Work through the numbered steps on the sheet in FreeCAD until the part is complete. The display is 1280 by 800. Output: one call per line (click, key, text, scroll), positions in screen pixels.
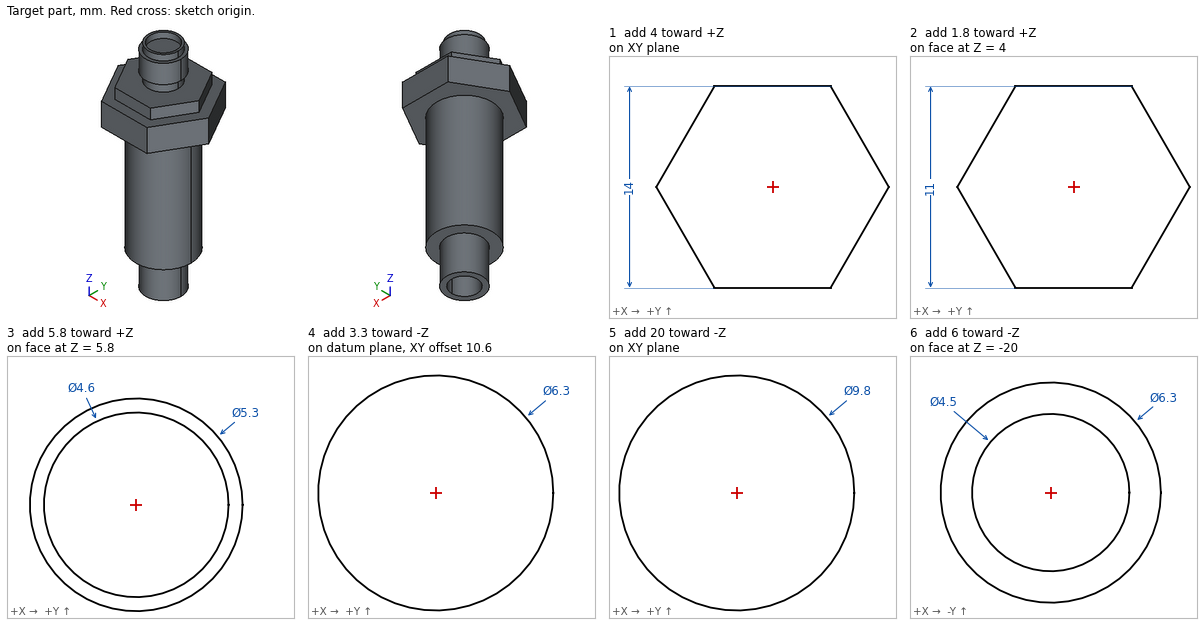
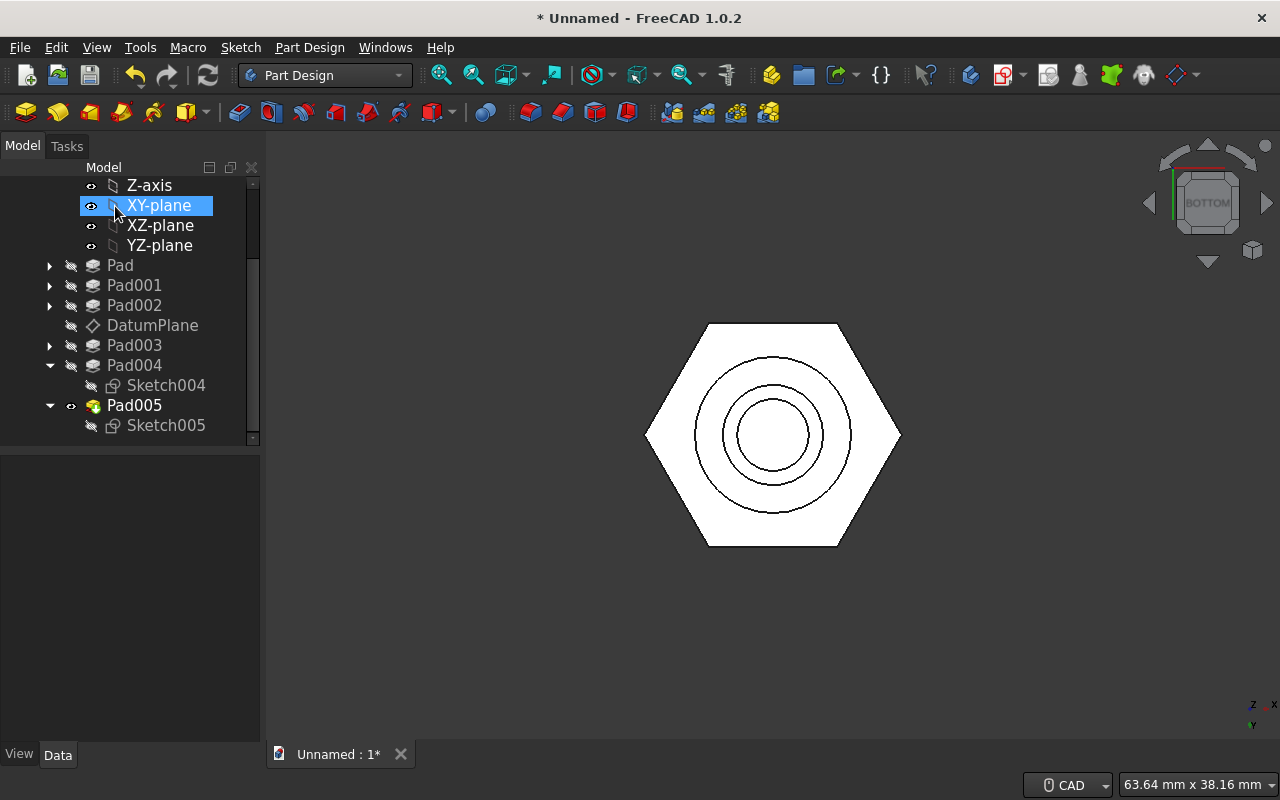
key(0)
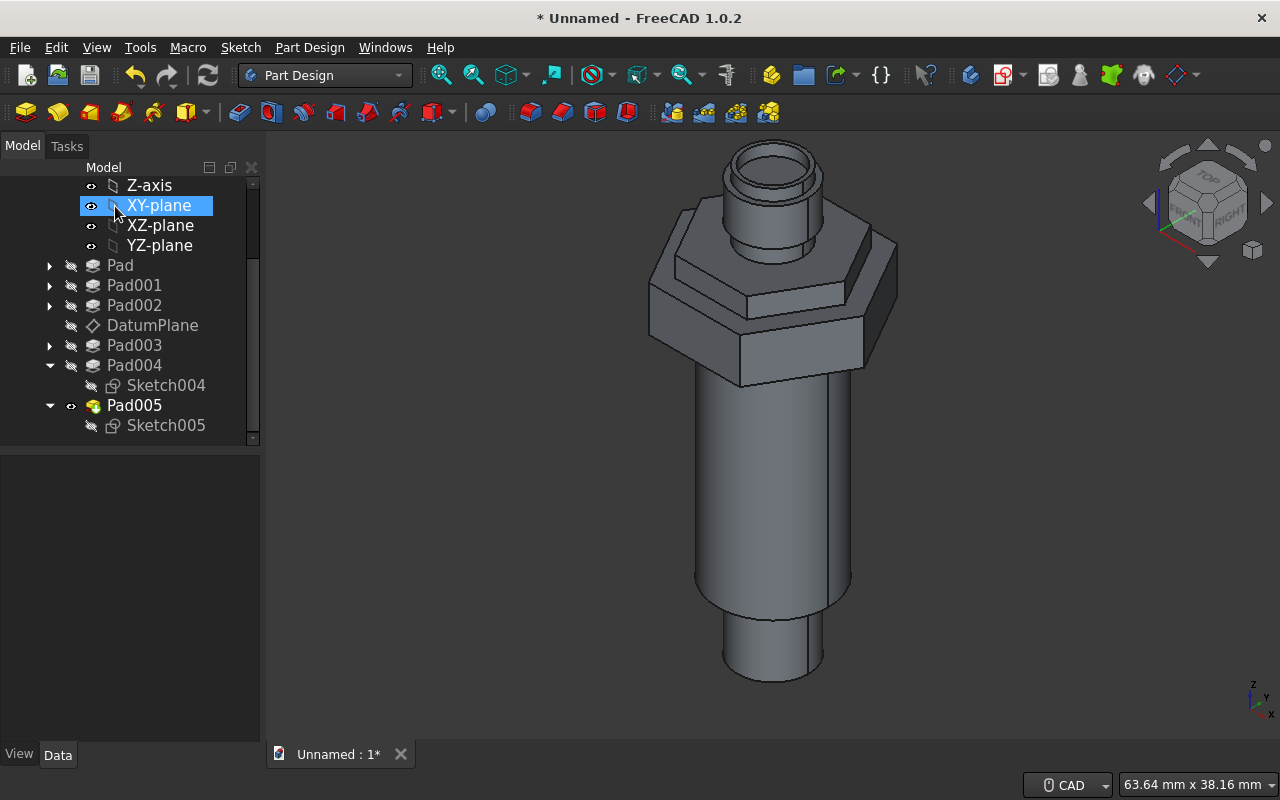
click(442, 76)